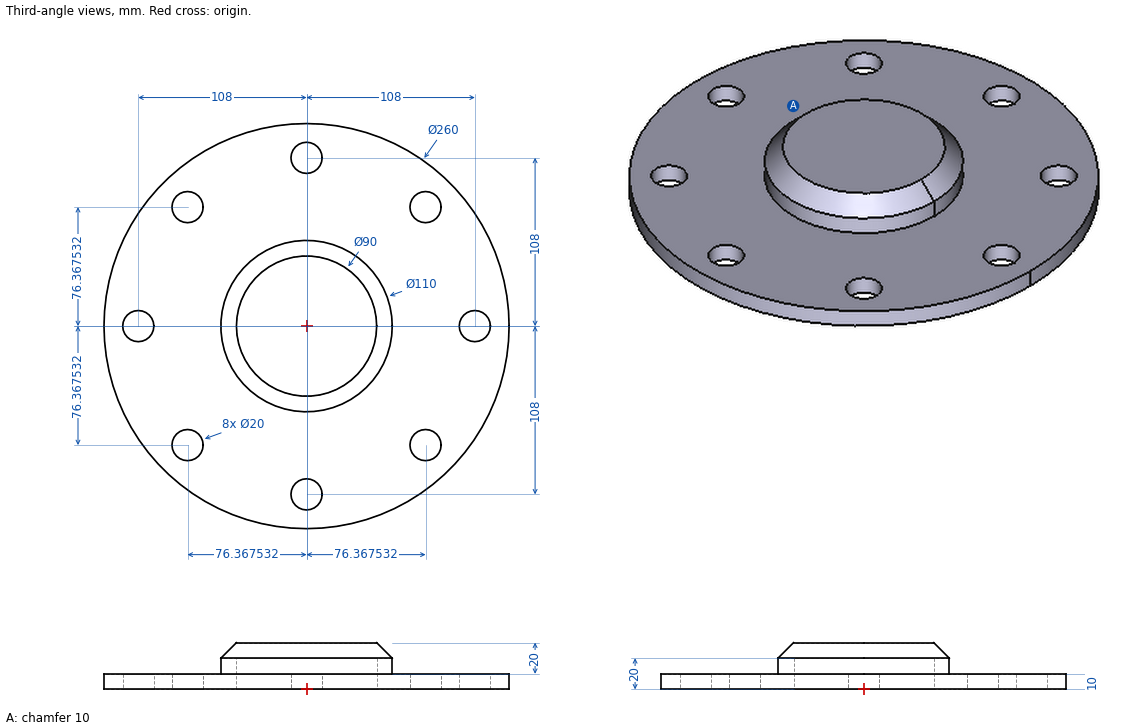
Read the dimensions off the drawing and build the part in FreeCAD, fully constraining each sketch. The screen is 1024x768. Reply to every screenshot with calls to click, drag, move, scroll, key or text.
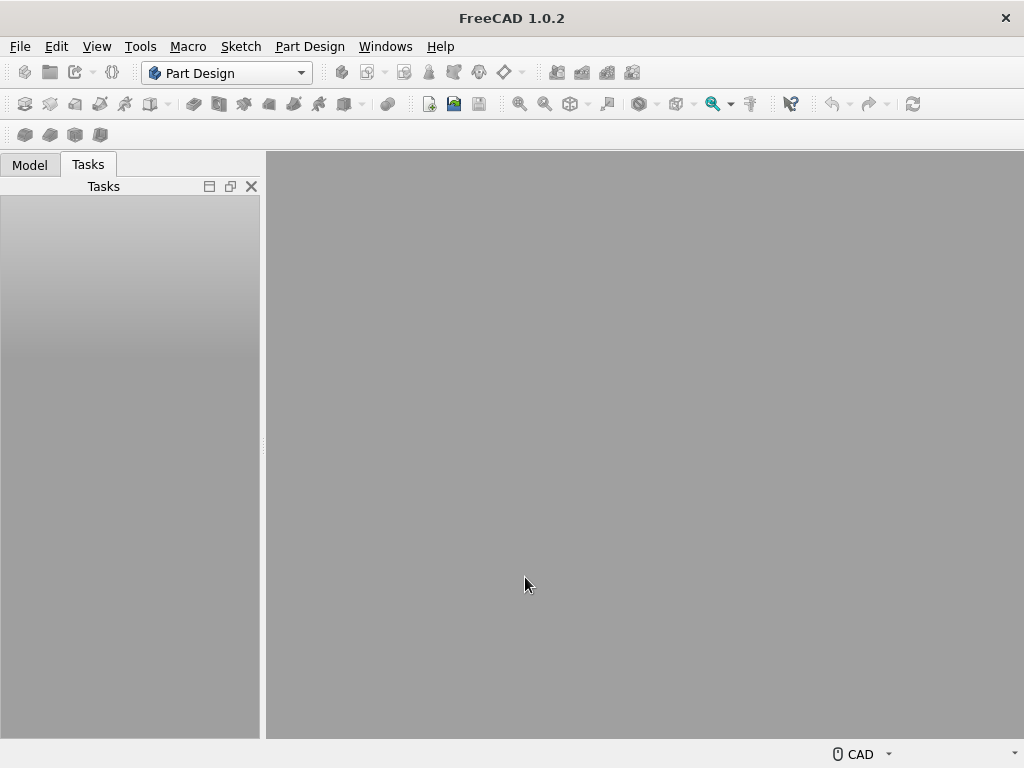
click(429, 104)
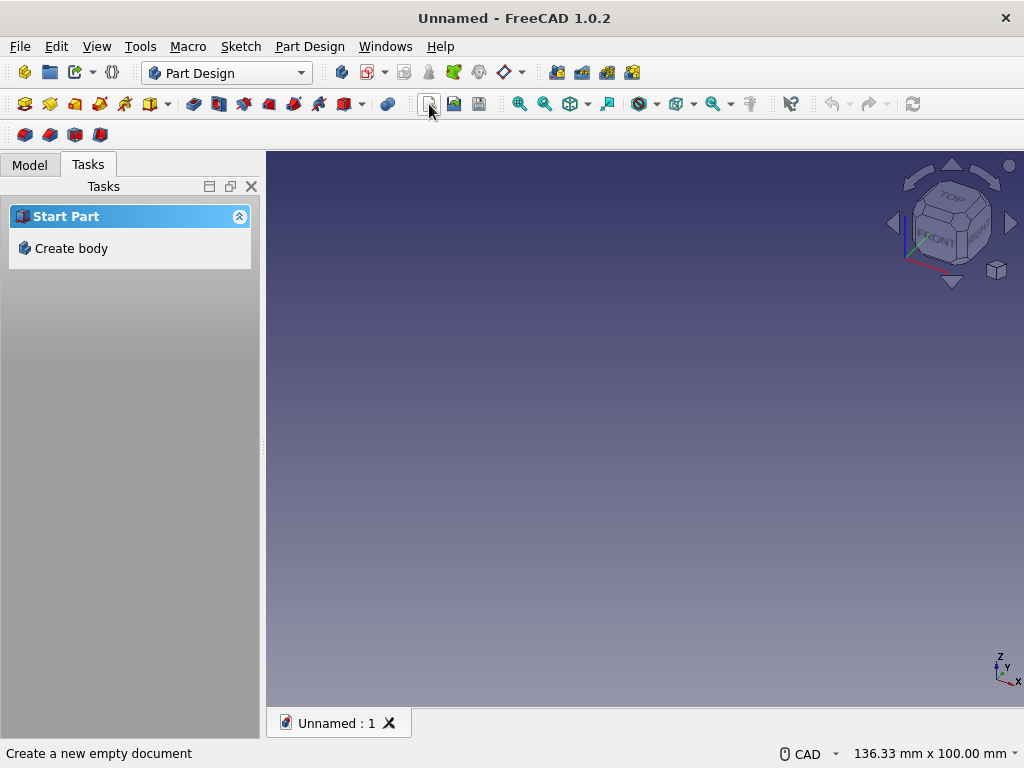
click(366, 72)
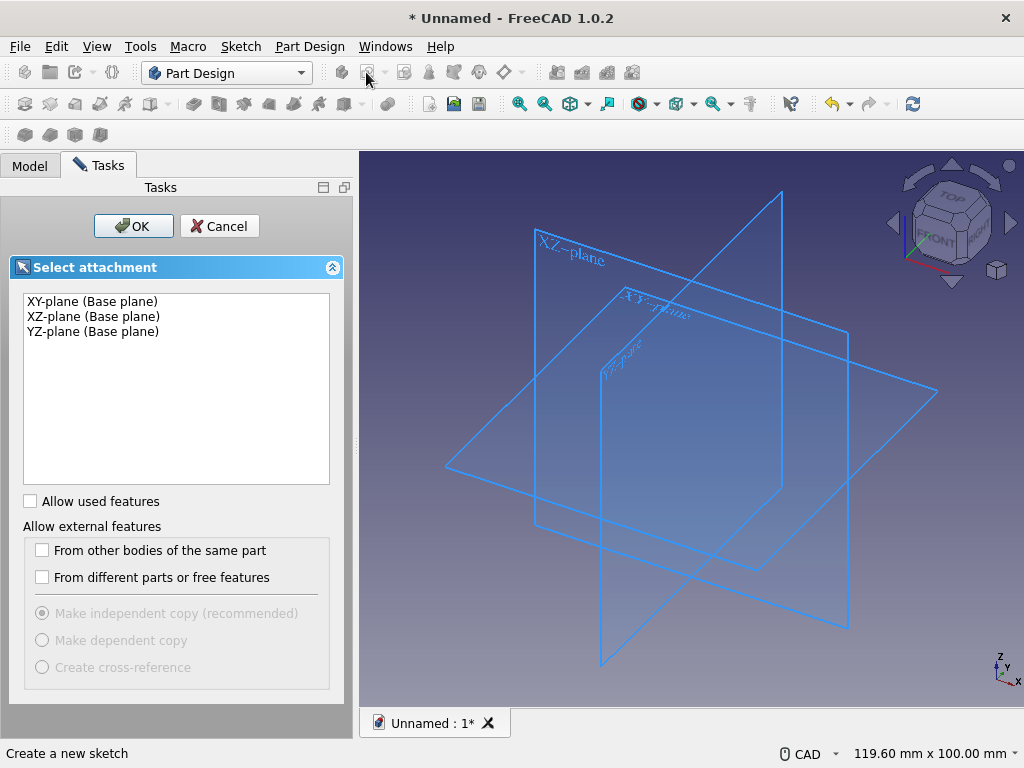
click(84, 302)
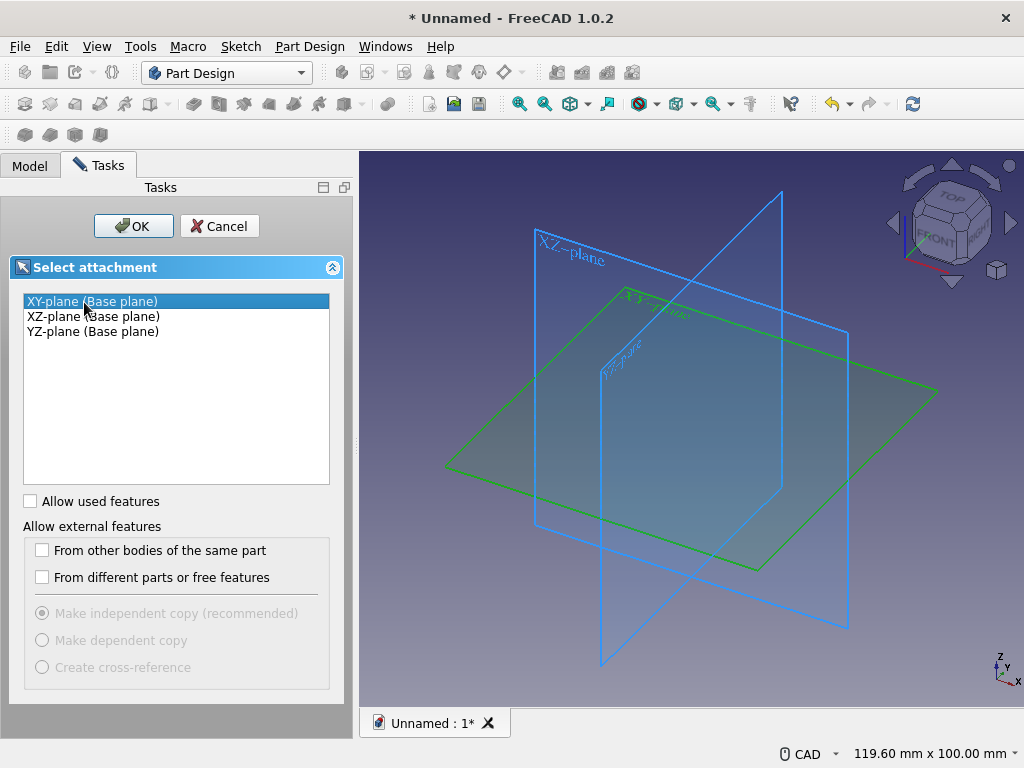
click(134, 226)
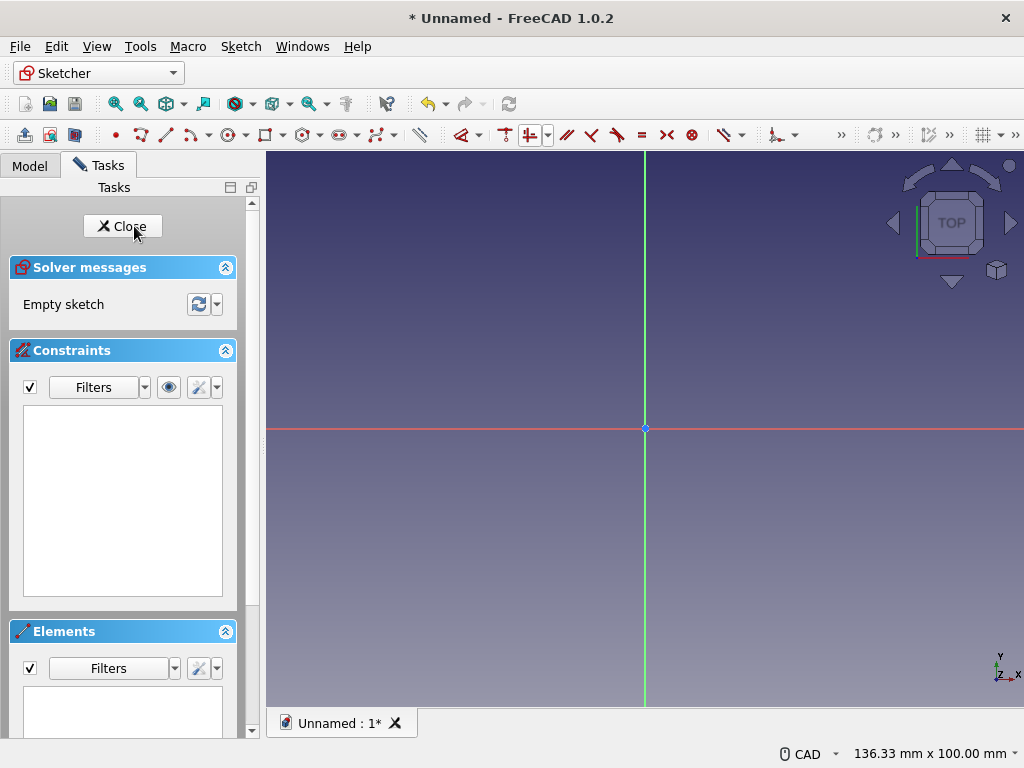
scroll(554, 429, down, 7)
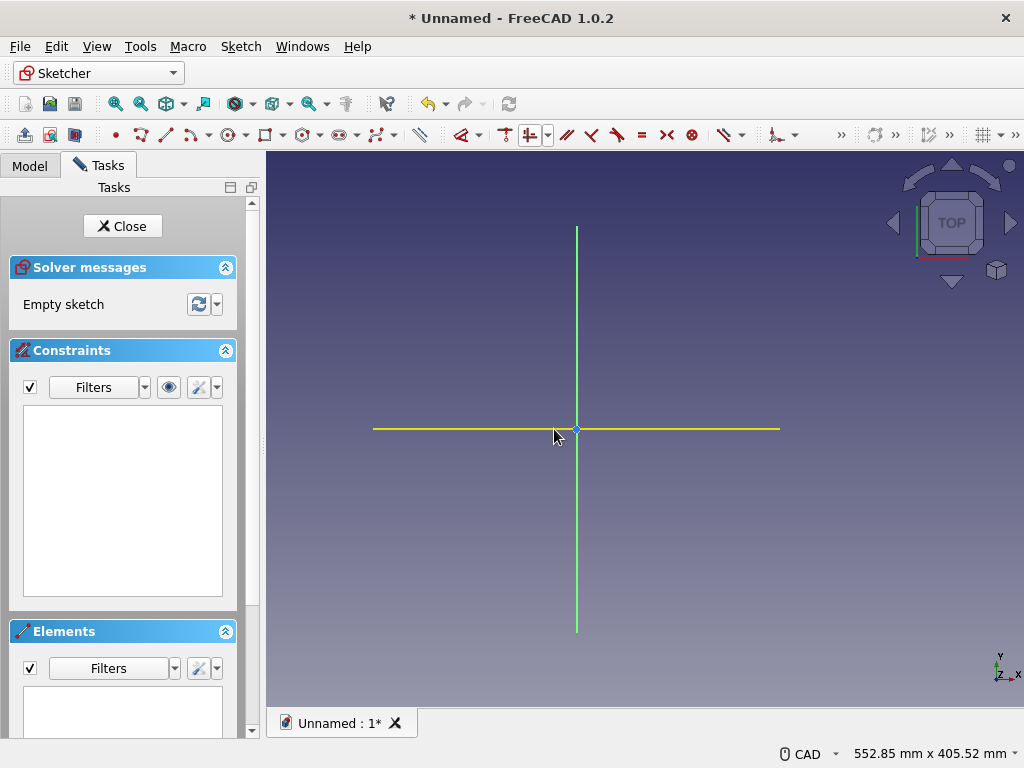
key(g)
key(c)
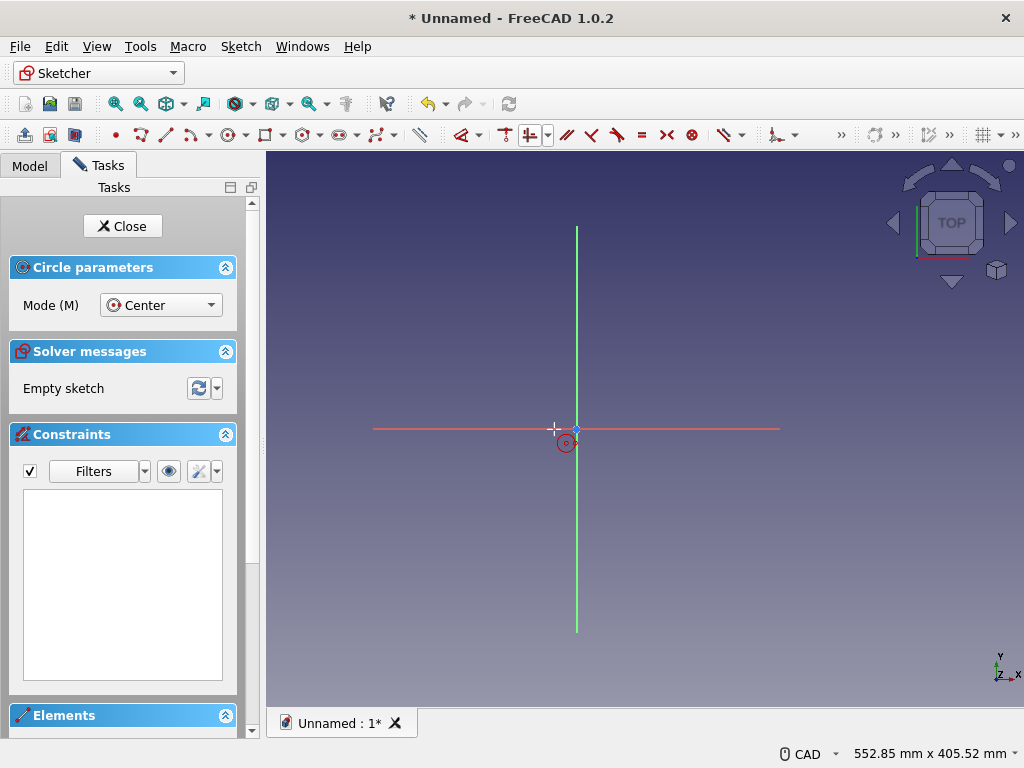
click(577, 429)
move(703, 303)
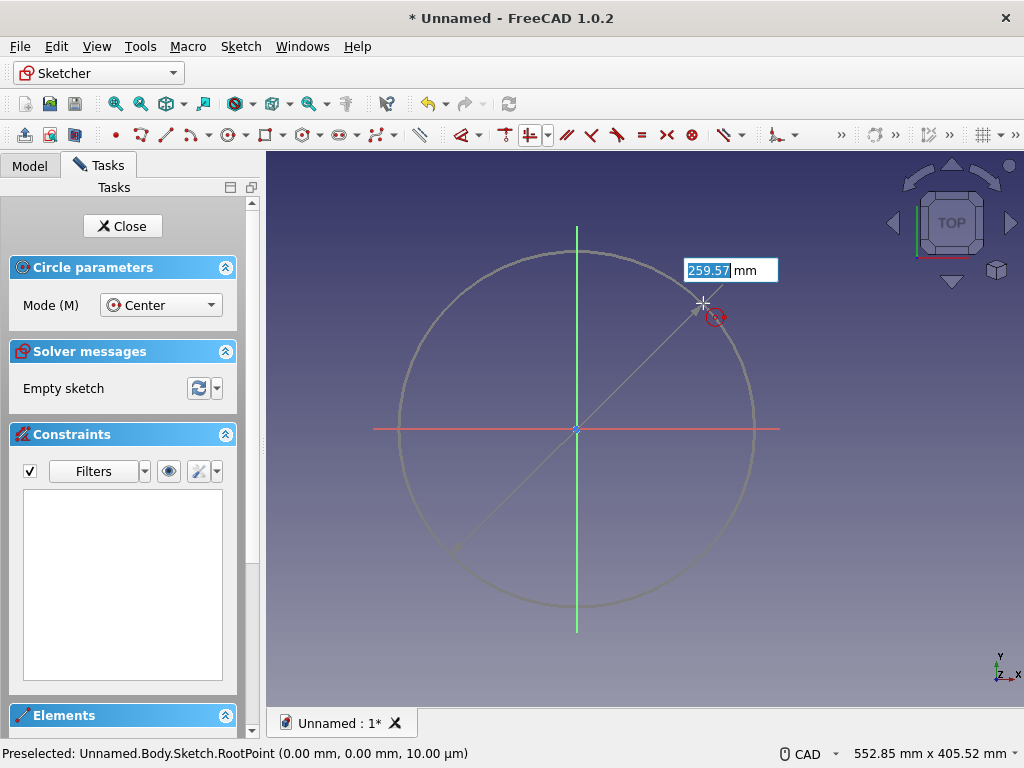
text(260)
key(Return)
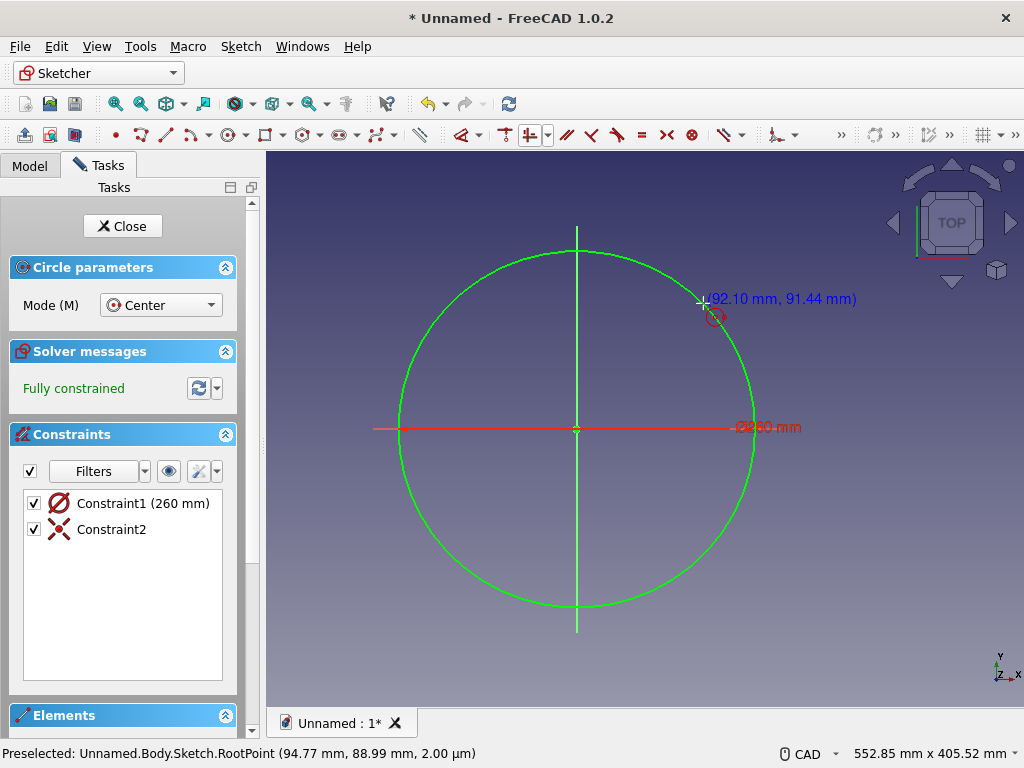
scroll(472, 534, up, 3)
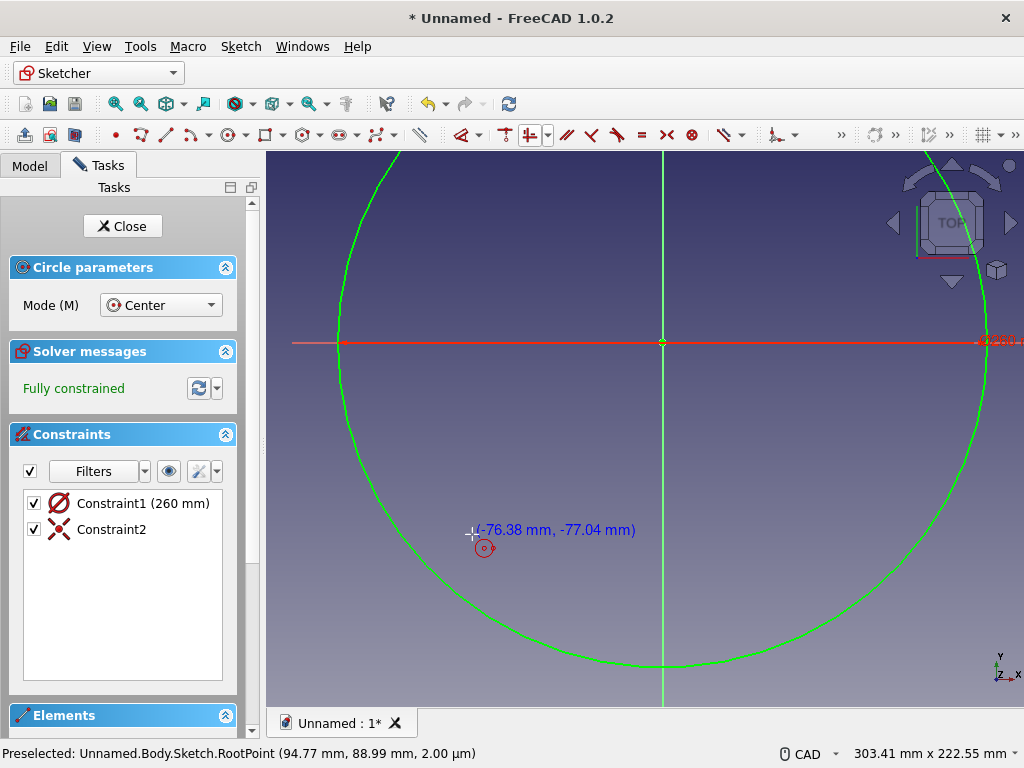
click(472, 534)
move(489, 516)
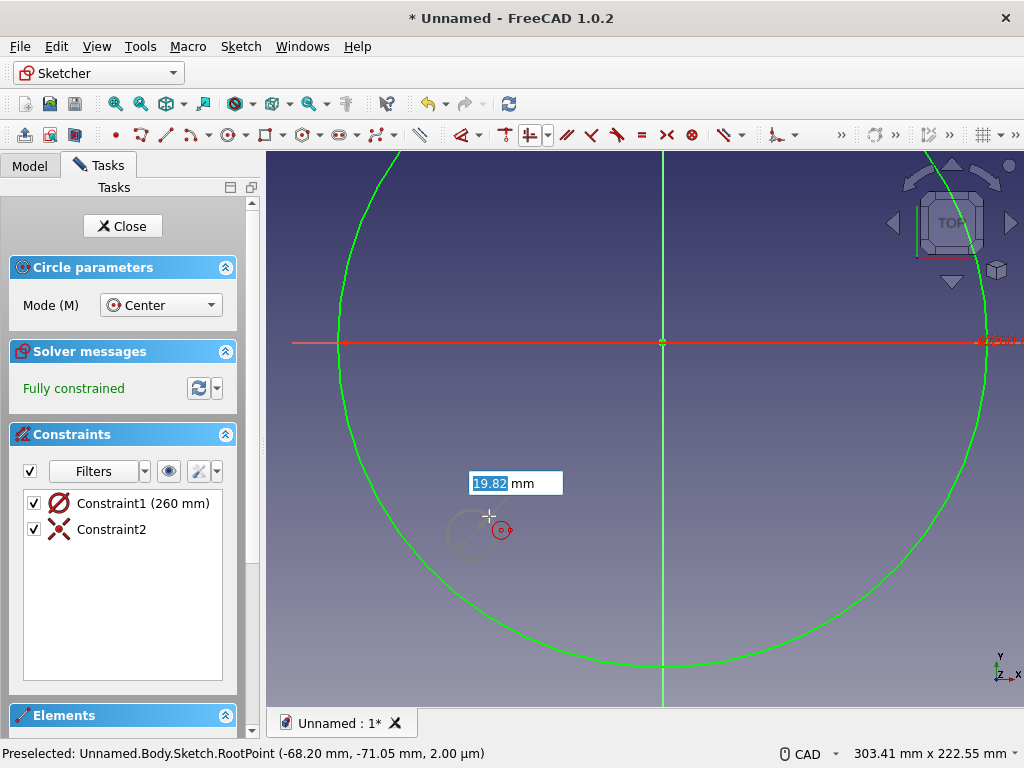
text(20)
key(Return)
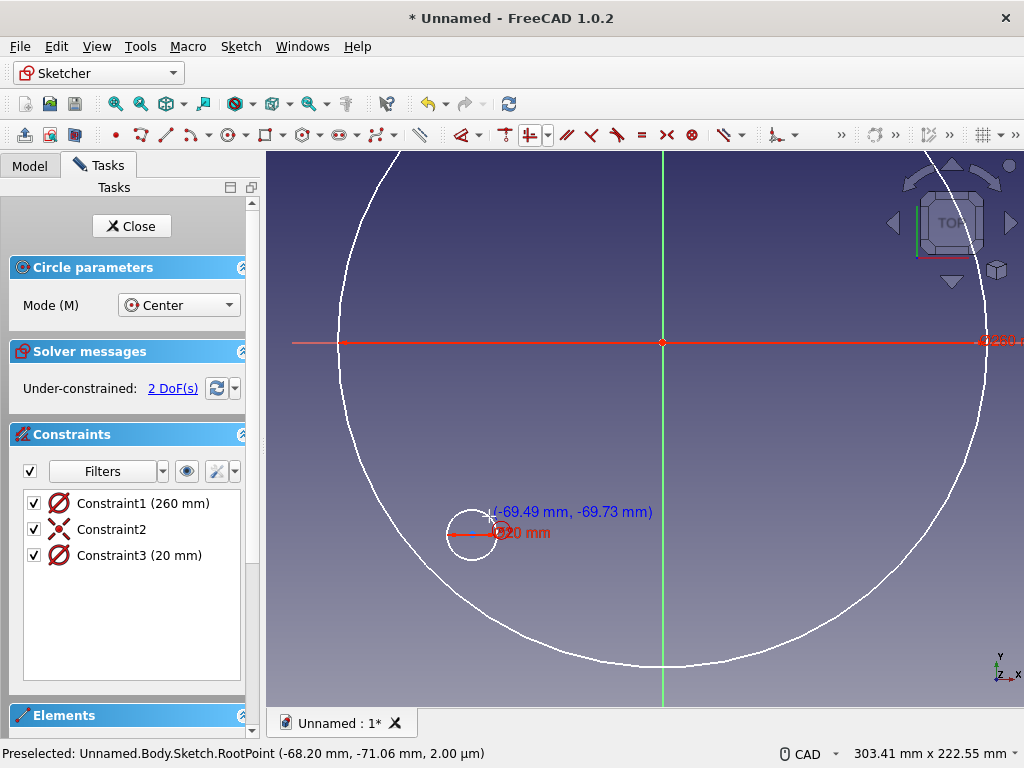
click(663, 613)
move(680, 595)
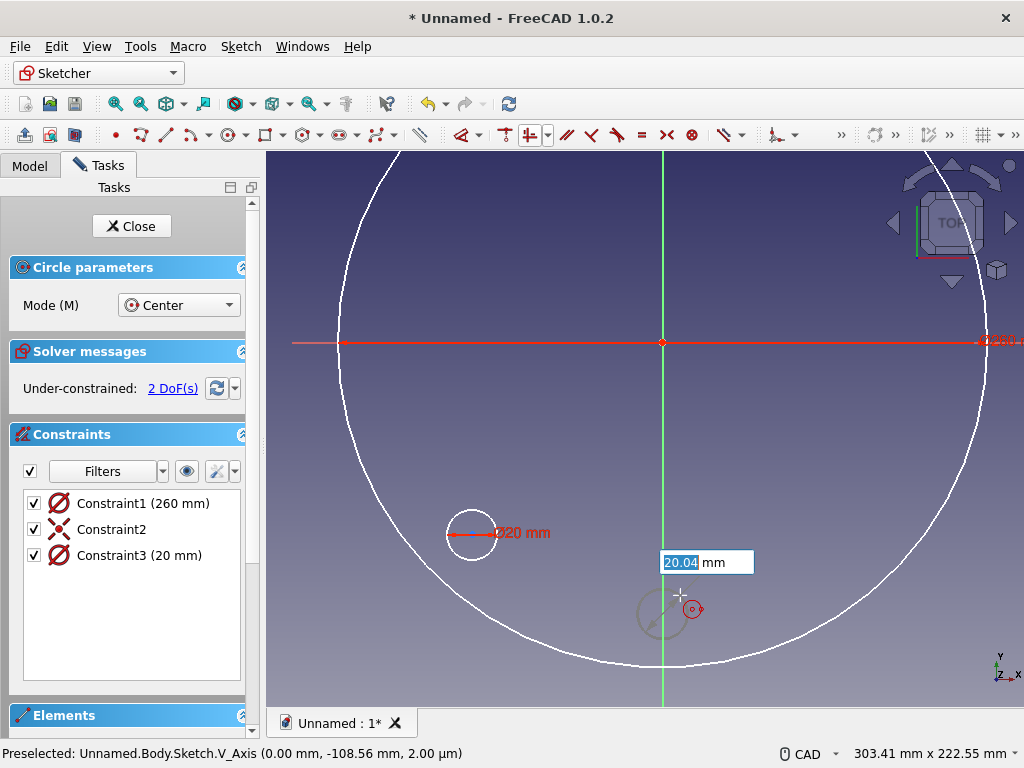
text(20)
key(Return)